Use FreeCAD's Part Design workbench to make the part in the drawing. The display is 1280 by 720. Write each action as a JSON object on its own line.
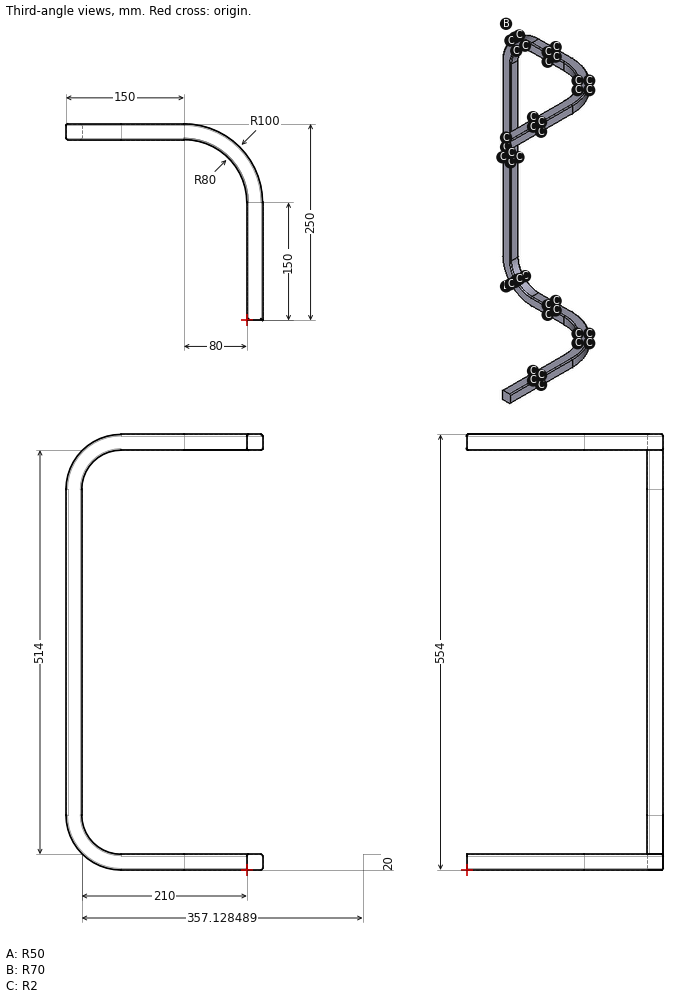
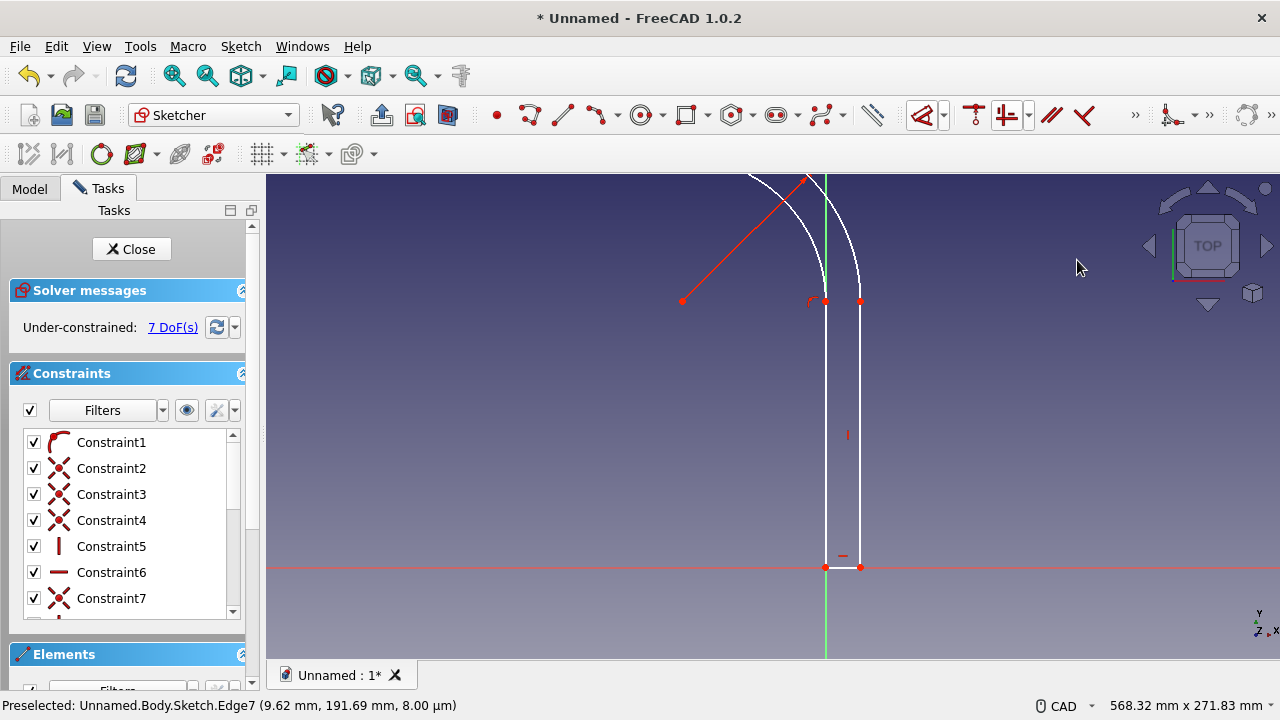
{"action": "left_click", "coordinate": [810, 236]}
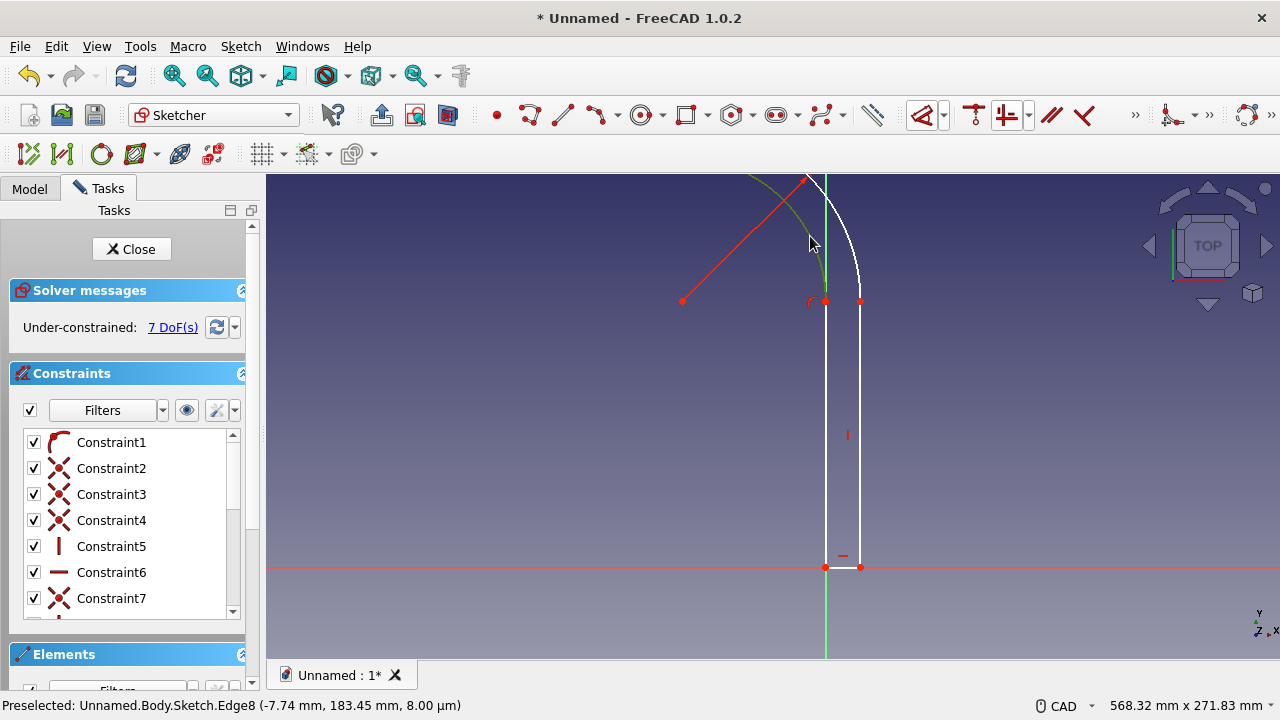
{"action": "left_click", "coordinate": [944, 116]}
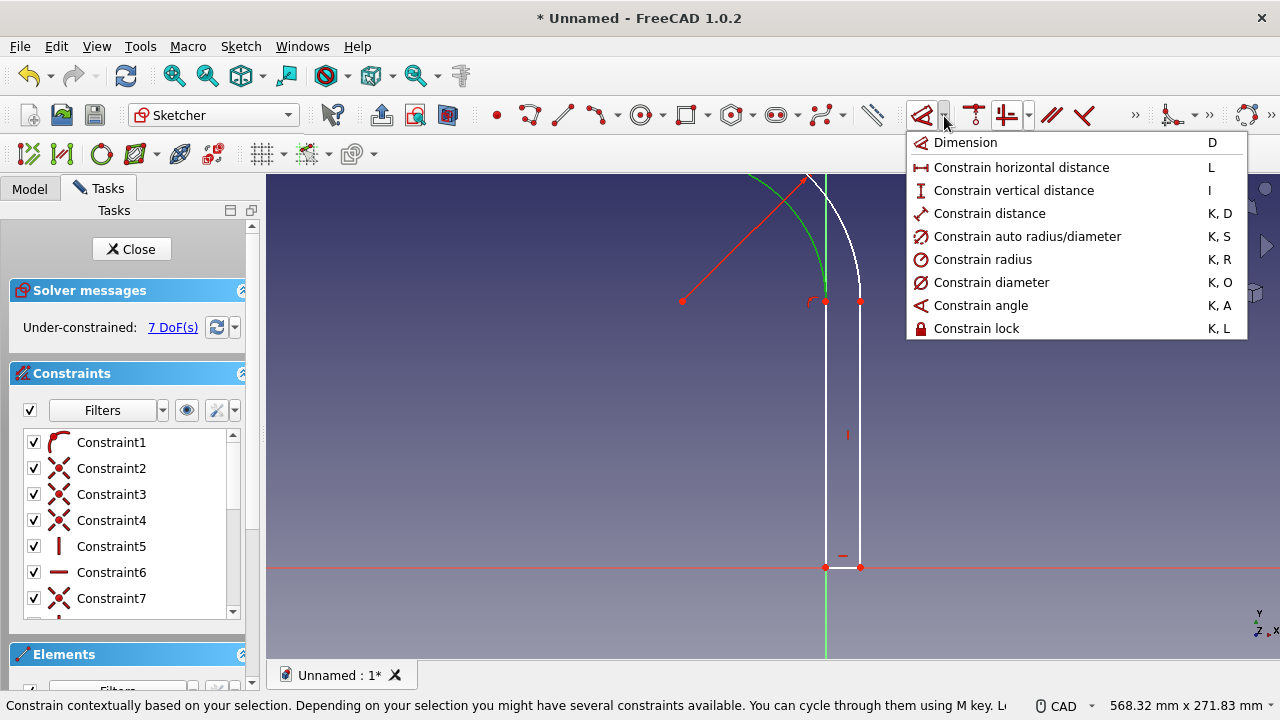
{"action": "left_click", "coordinate": [1077, 260]}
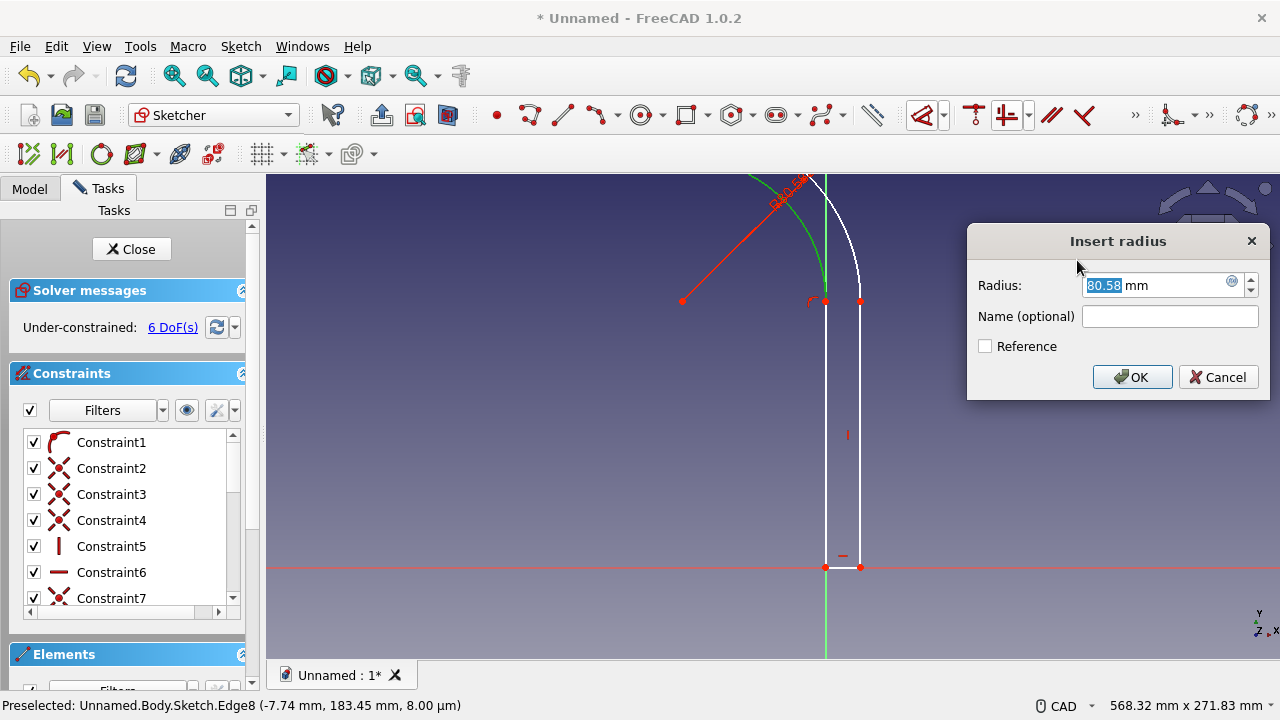
{"action": "type", "text": "80"}
{"action": "key", "text": "Return"}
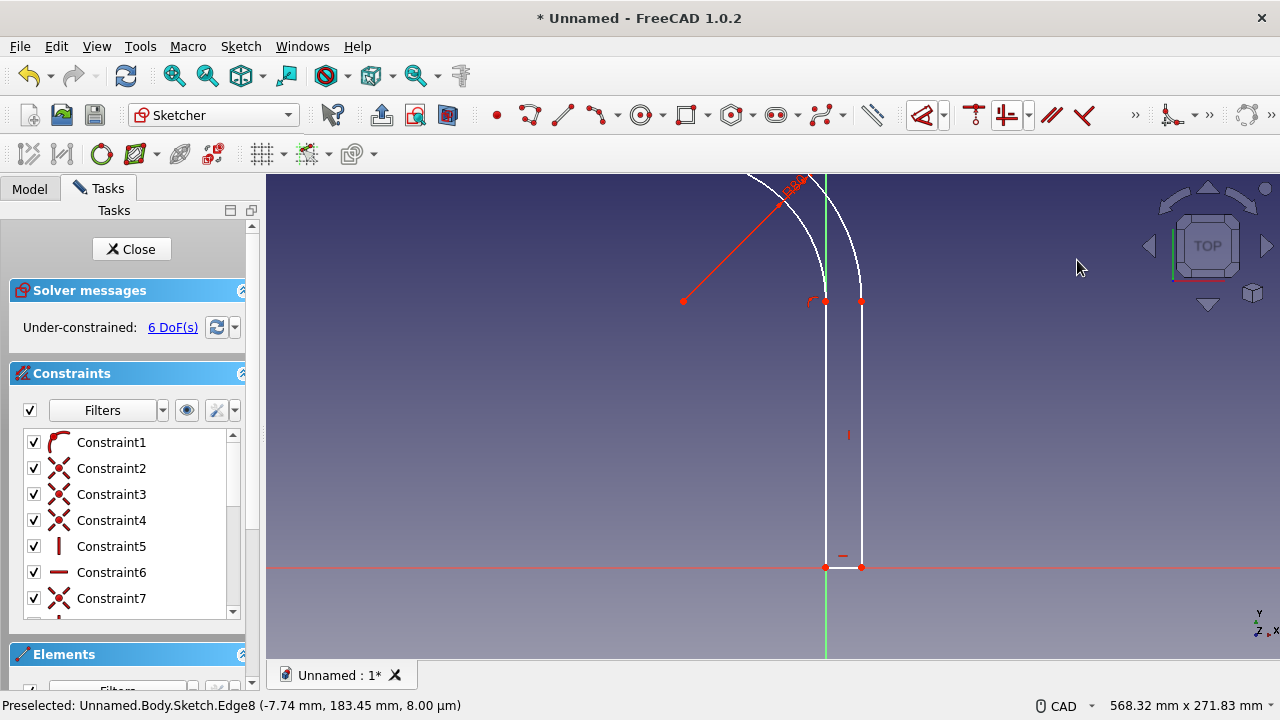
{"action": "left_click", "coordinate": [826, 381]}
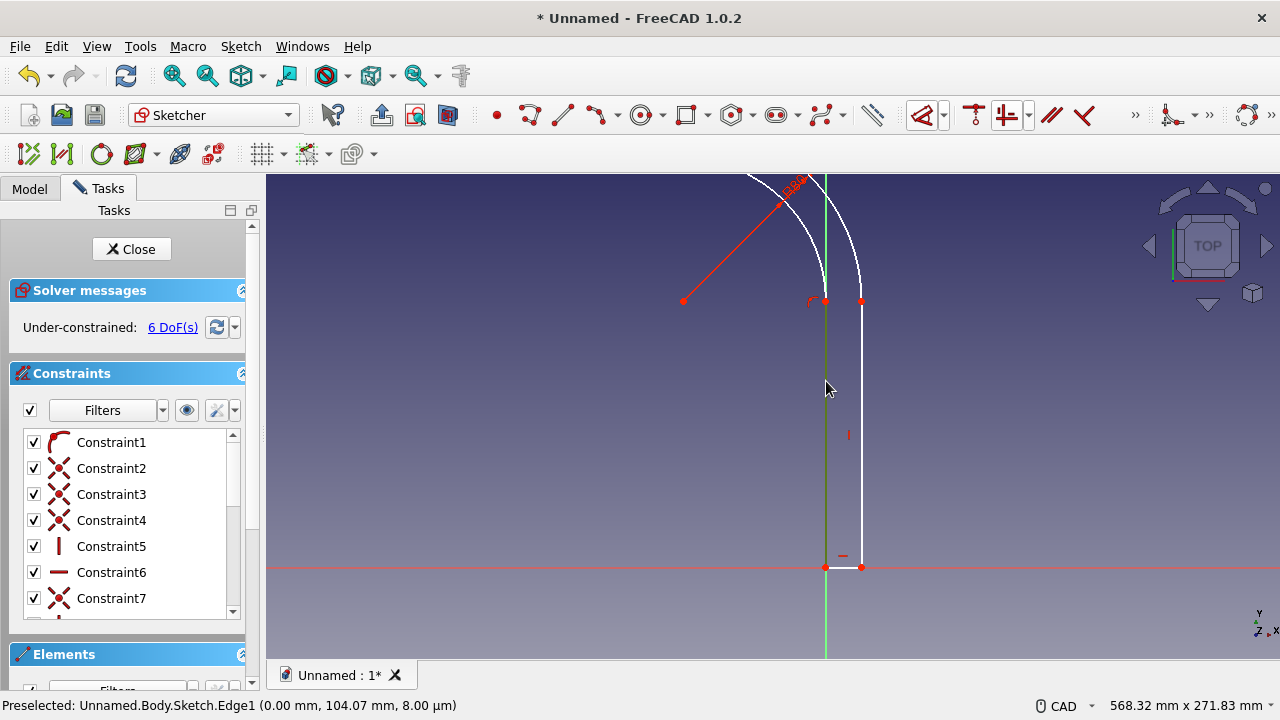
{"action": "left_click", "coordinate": [944, 116]}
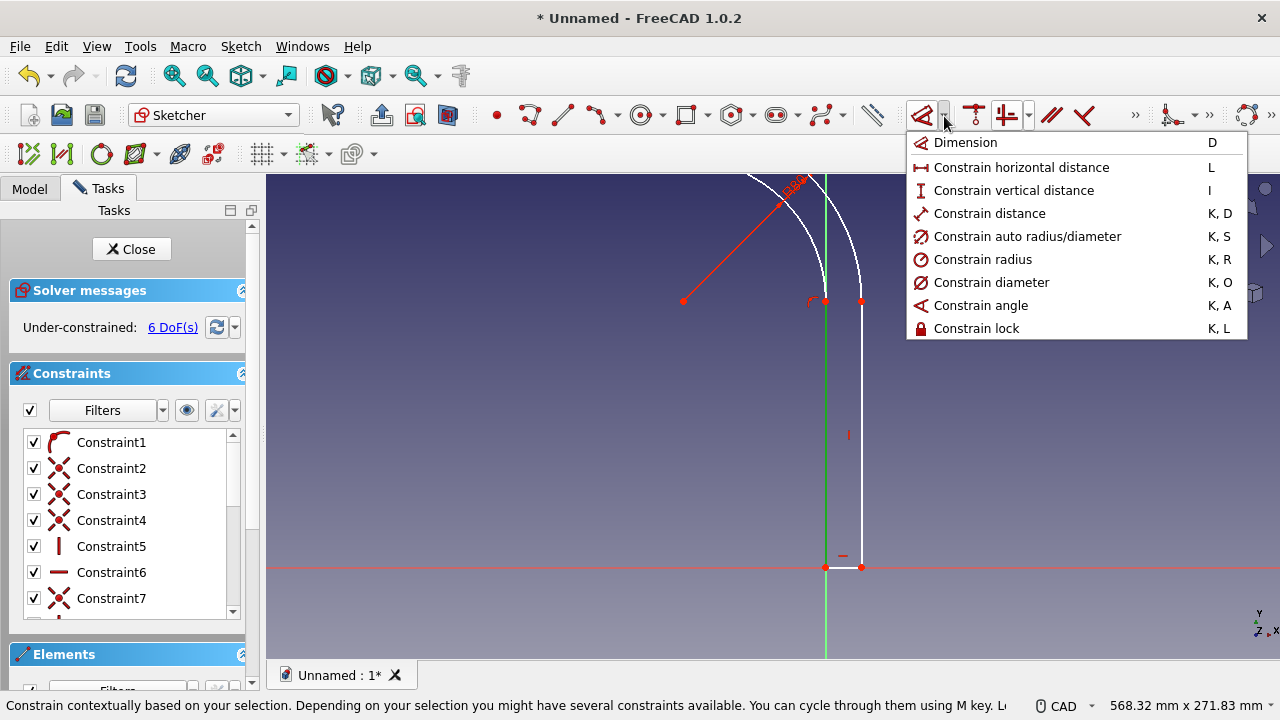
{"action": "left_click", "coordinate": [1077, 190]}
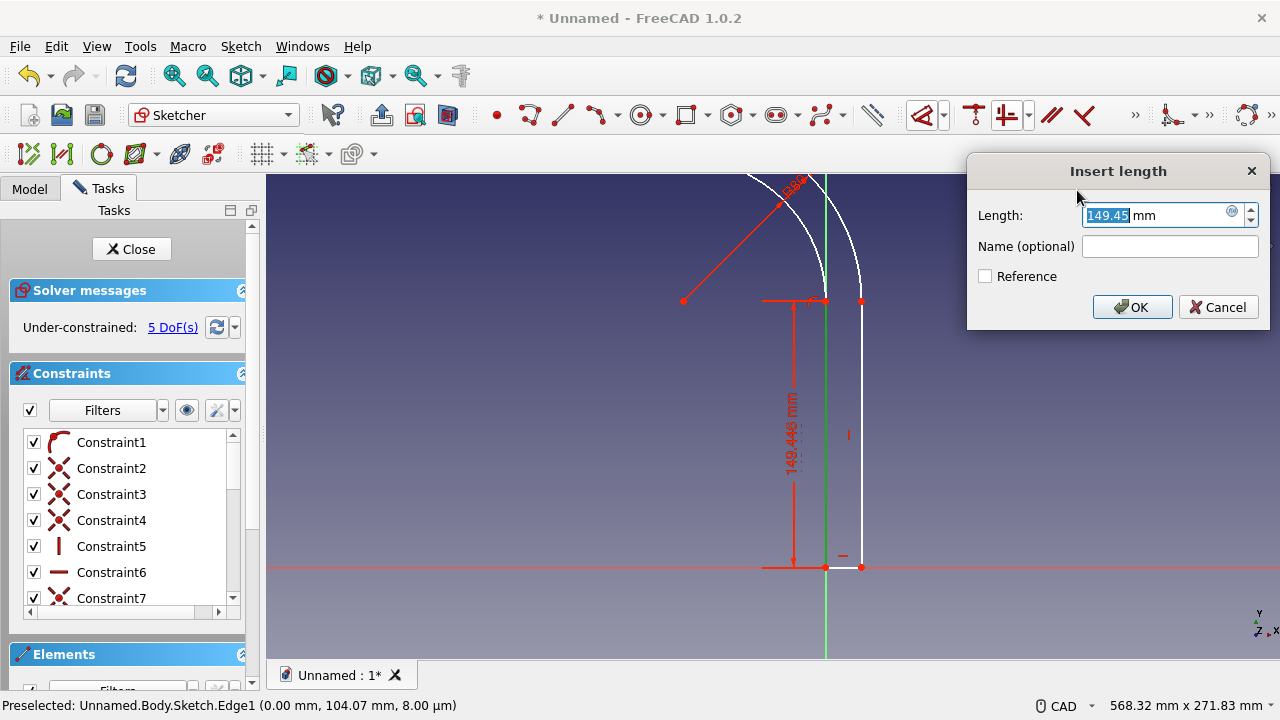
{"action": "type", "text": "150"}
{"action": "key", "text": "Return"}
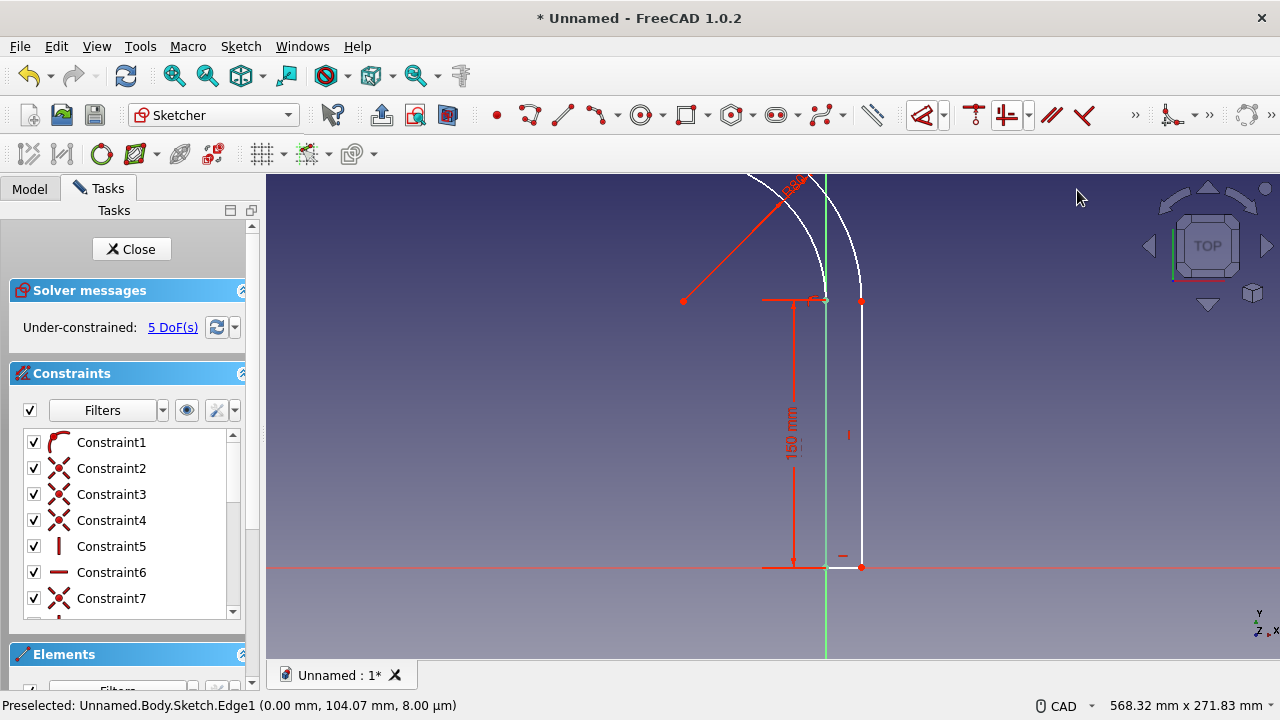
{"action": "left_click", "coordinate": [862, 488]}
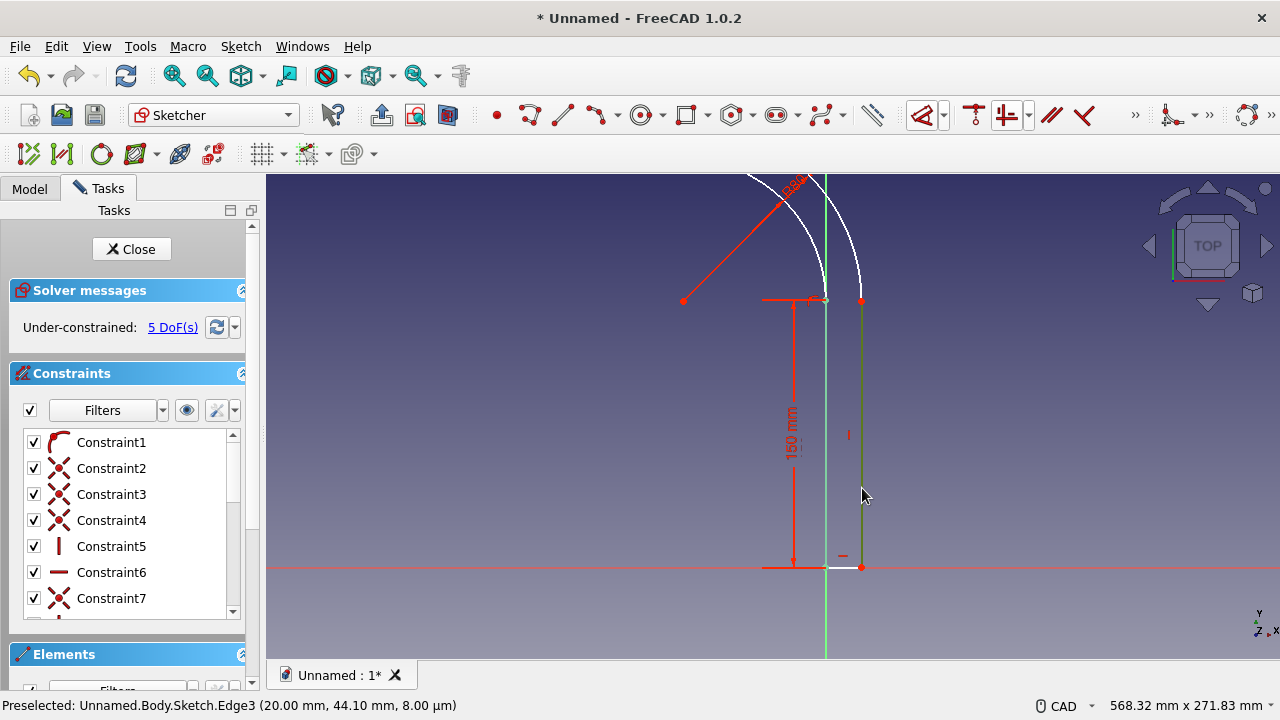
{"action": "key", "text": "i"}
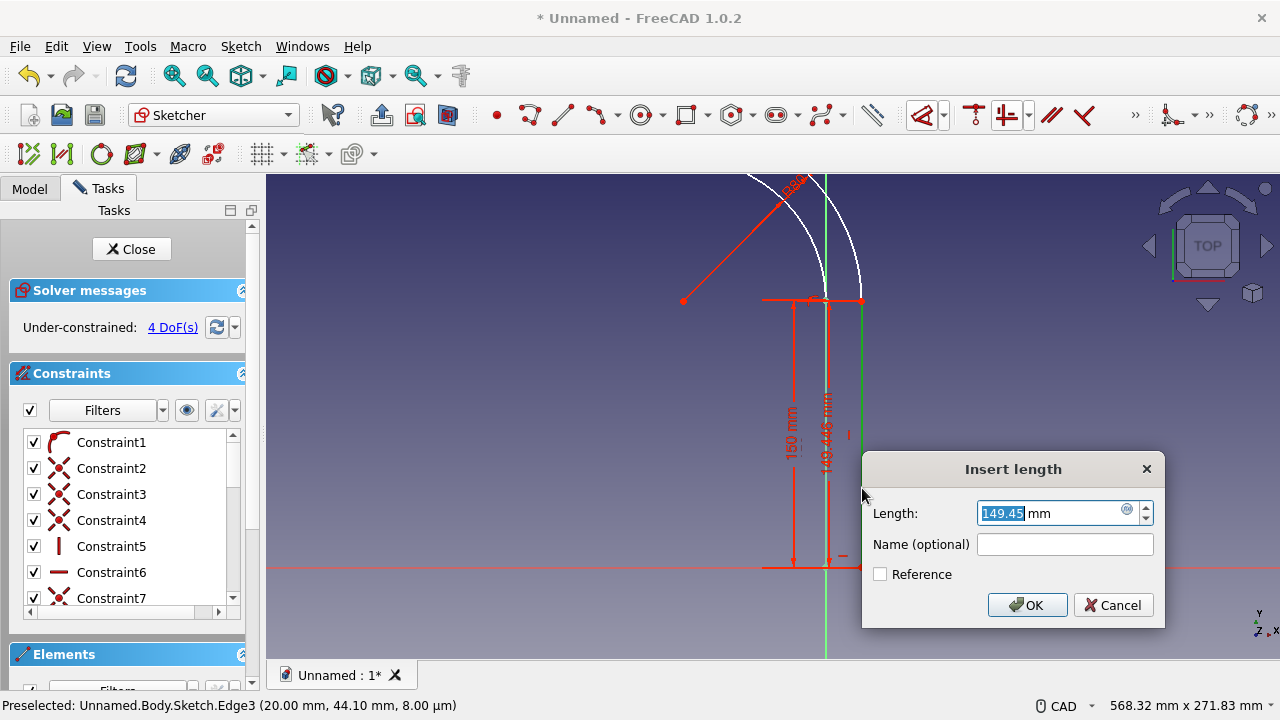
{"action": "type", "text": "150"}
{"action": "key", "text": "Return"}